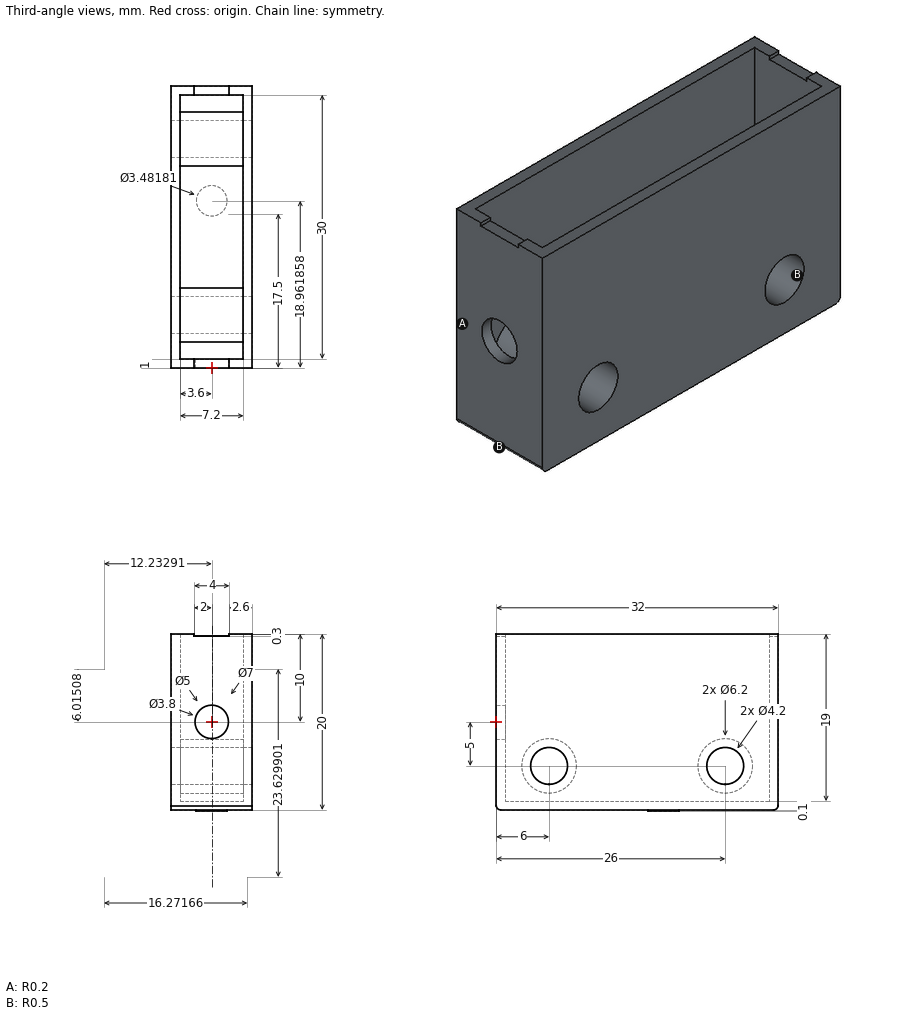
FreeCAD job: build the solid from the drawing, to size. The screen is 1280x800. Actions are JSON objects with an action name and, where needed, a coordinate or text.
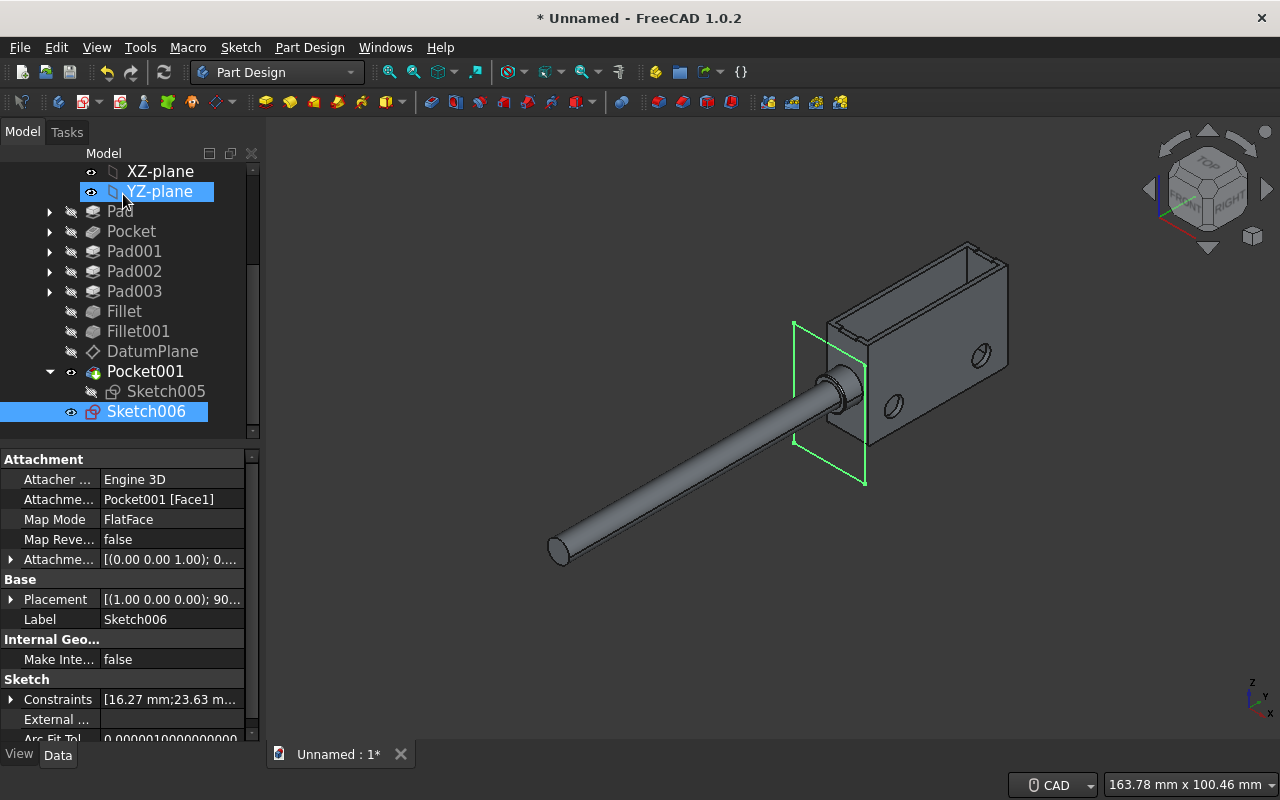
{"action": "left_click", "coordinate": [432, 102]}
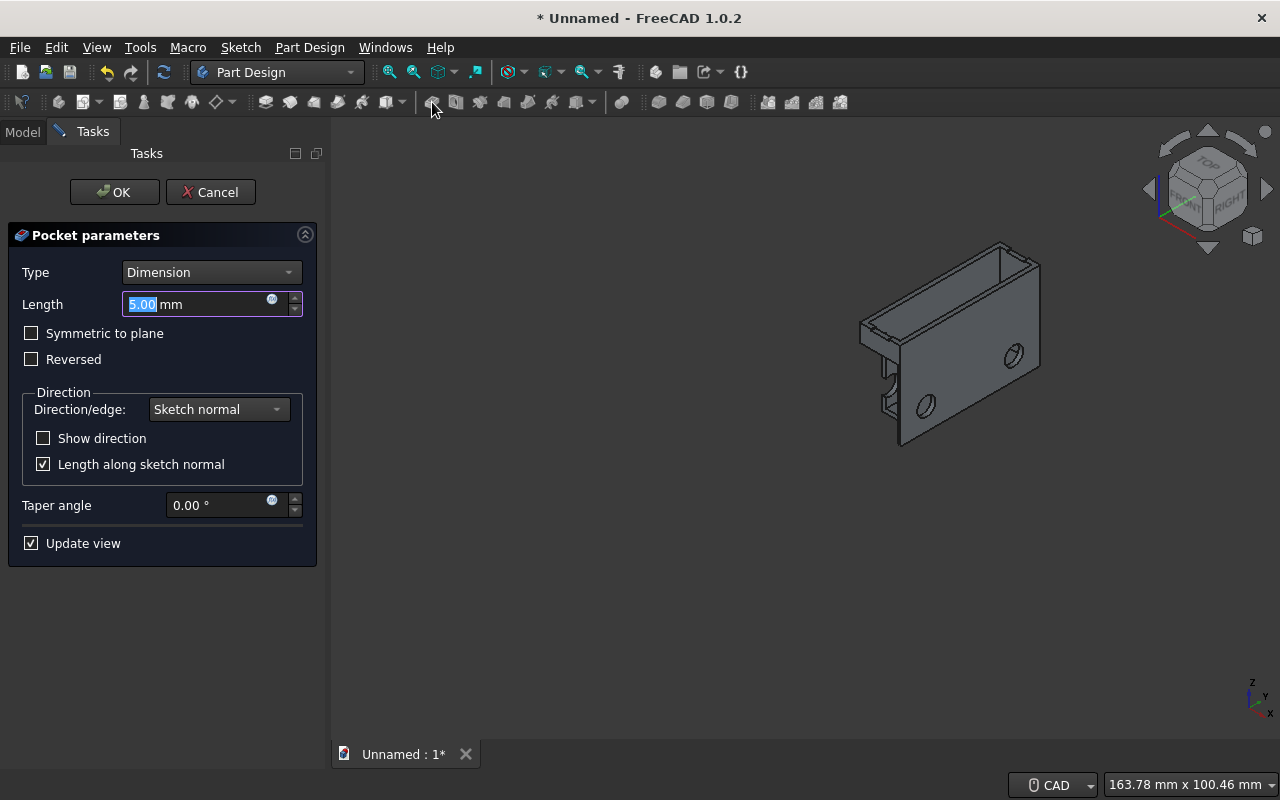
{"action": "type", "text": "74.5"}
{"action": "key", "text": "Tab"}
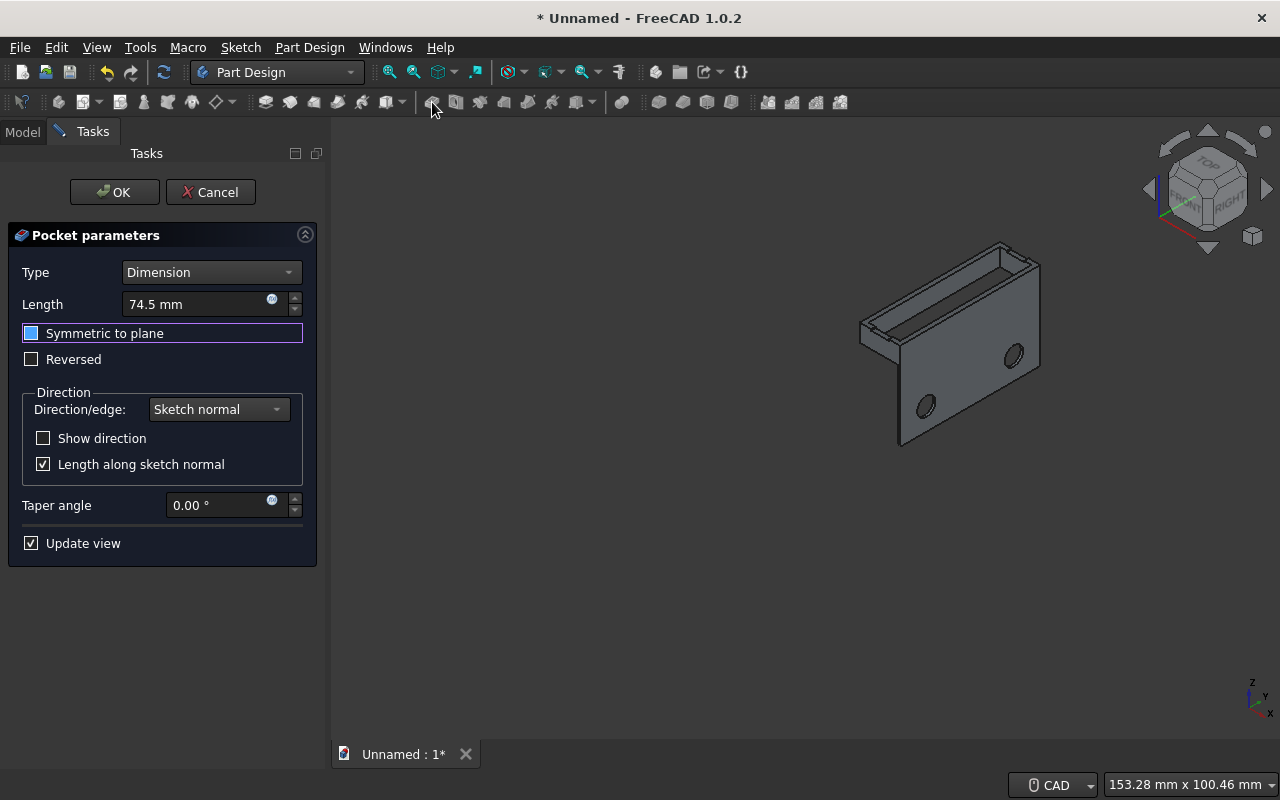
{"action": "left_click", "coordinate": [30, 359]}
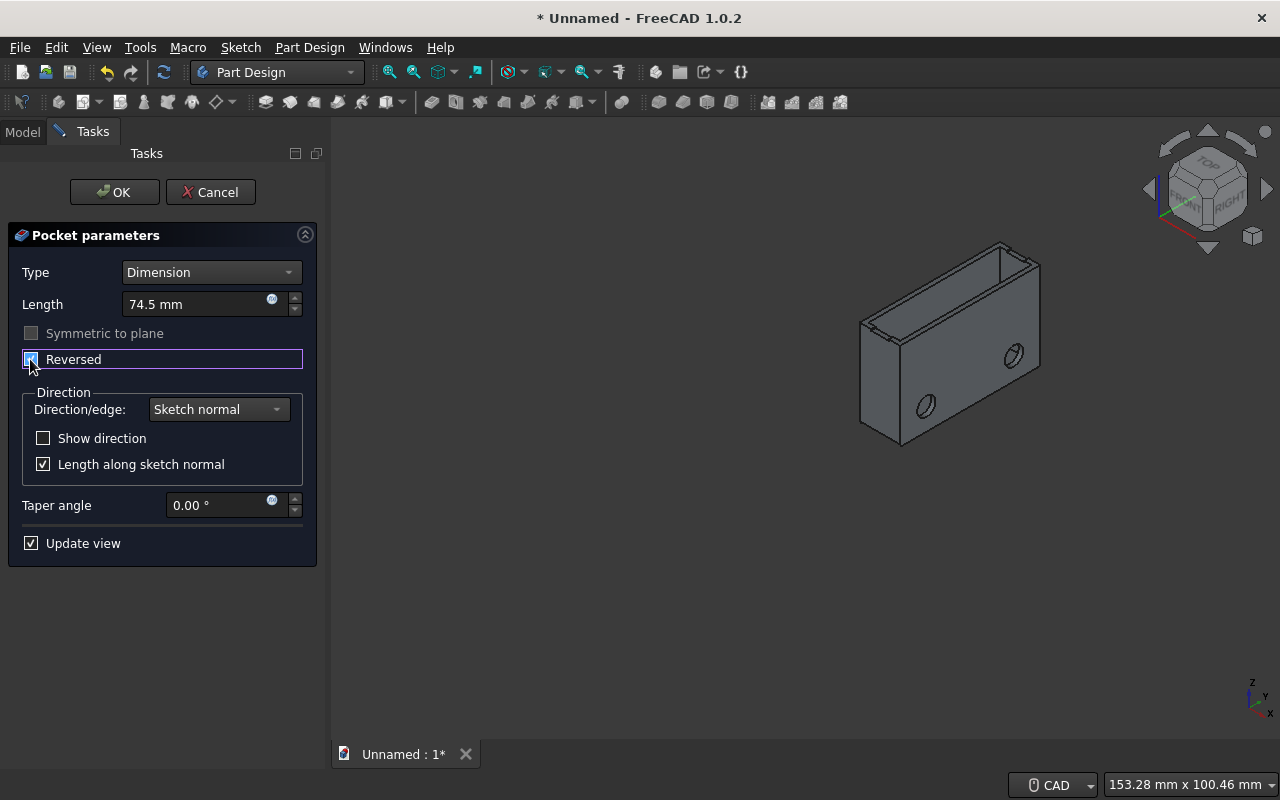
{"action": "left_click", "coordinate": [115, 192]}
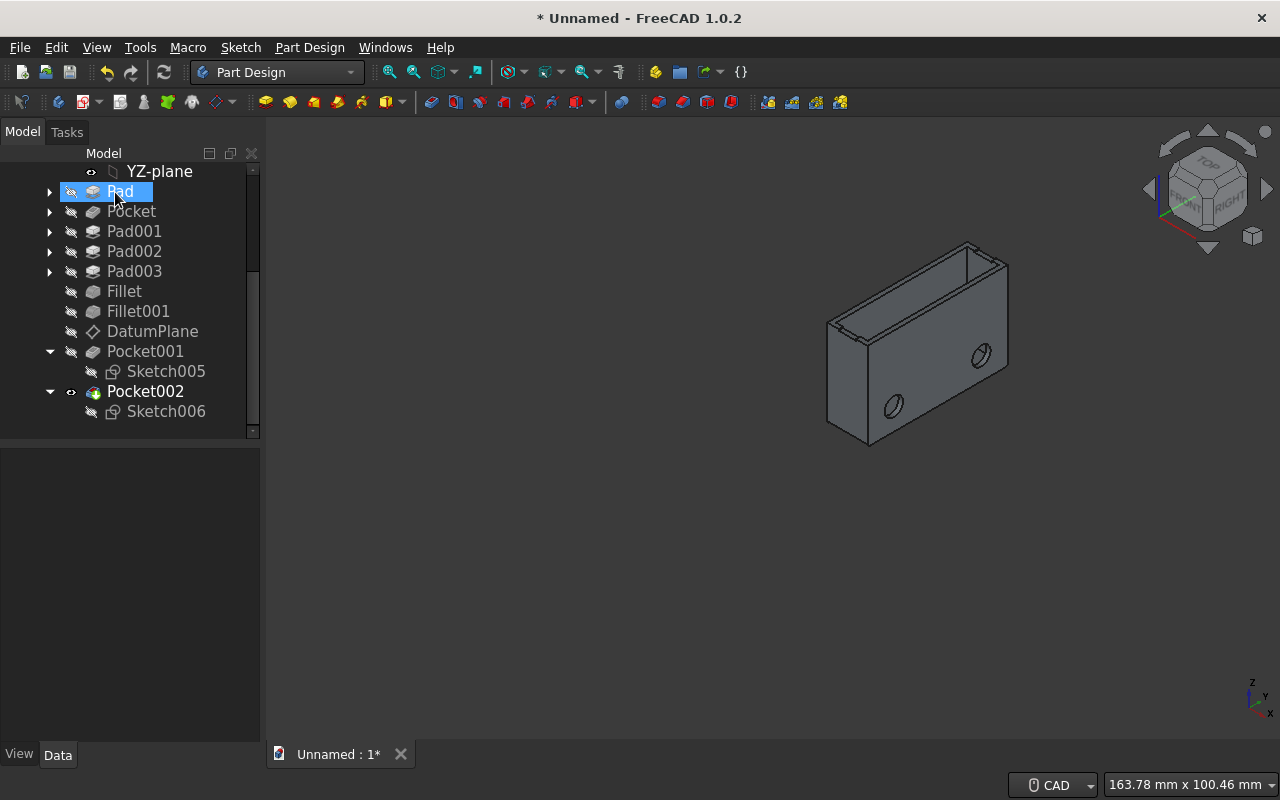
{"action": "left_click", "coordinate": [390, 72]}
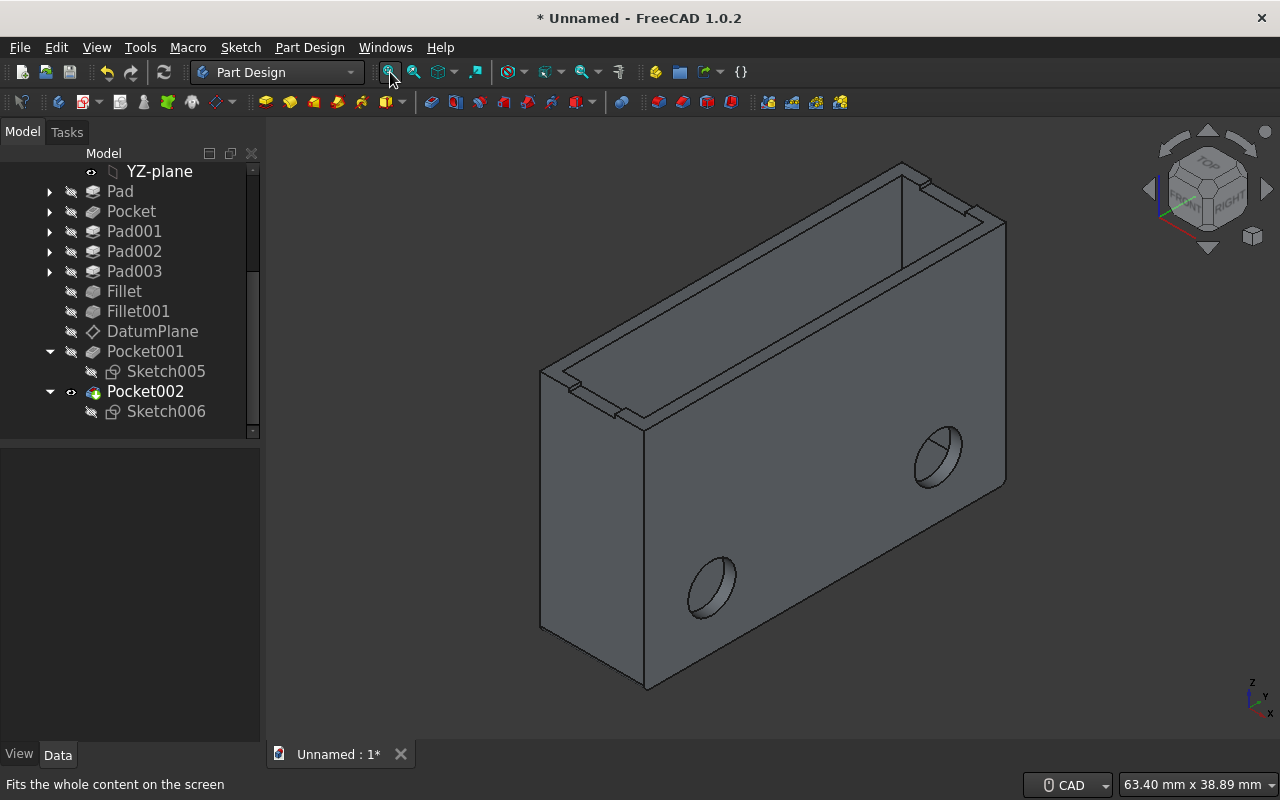
{"action": "left_click", "coordinate": [592, 491]}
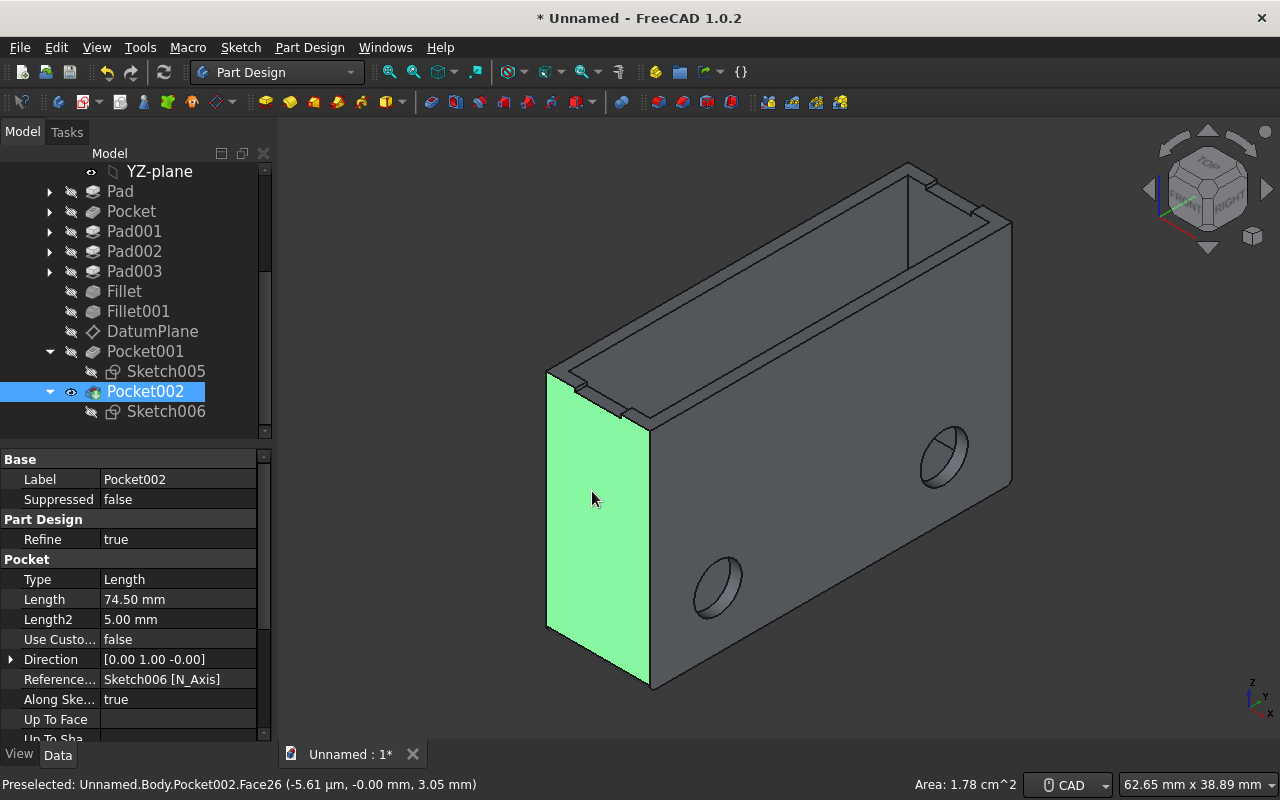
{"action": "left_click", "coordinate": [84, 102]}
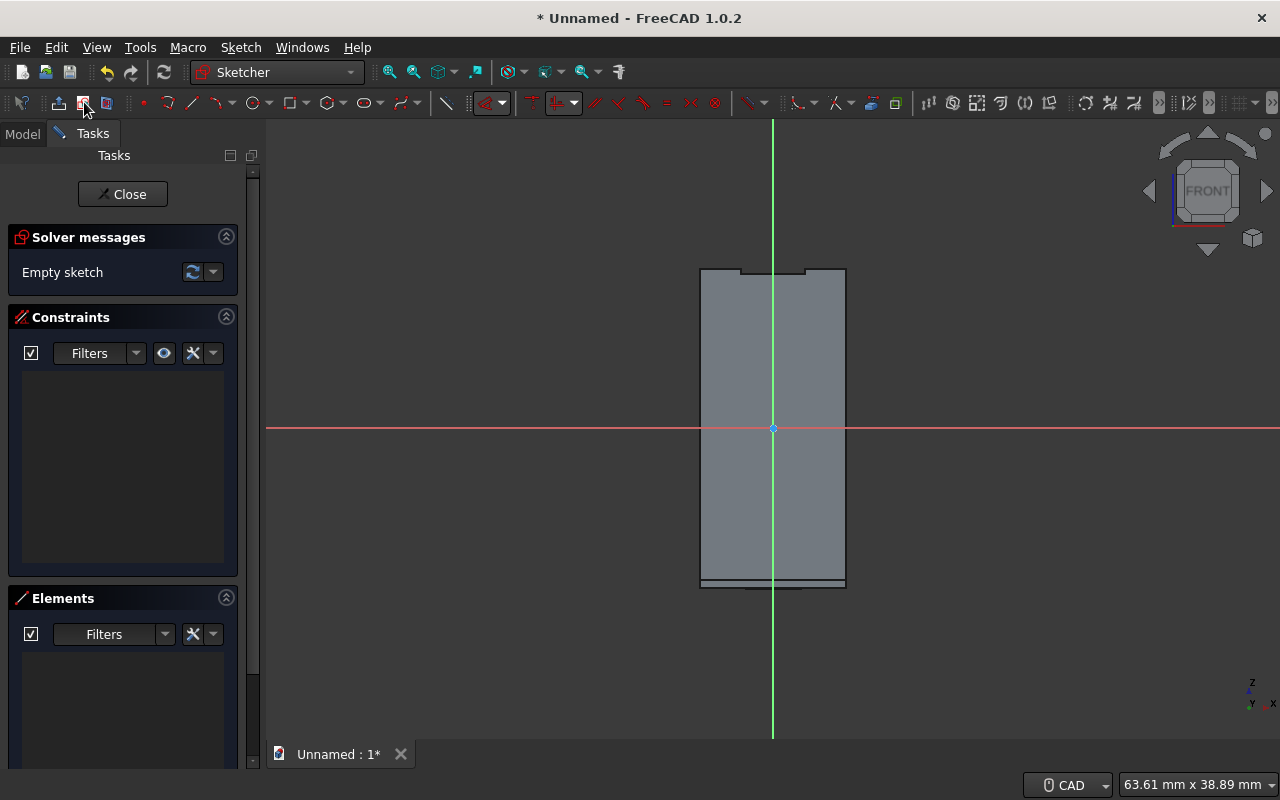
{"action": "scroll", "coordinate": [787, 428], "scroll_direction": "up", "scroll_amount": 9}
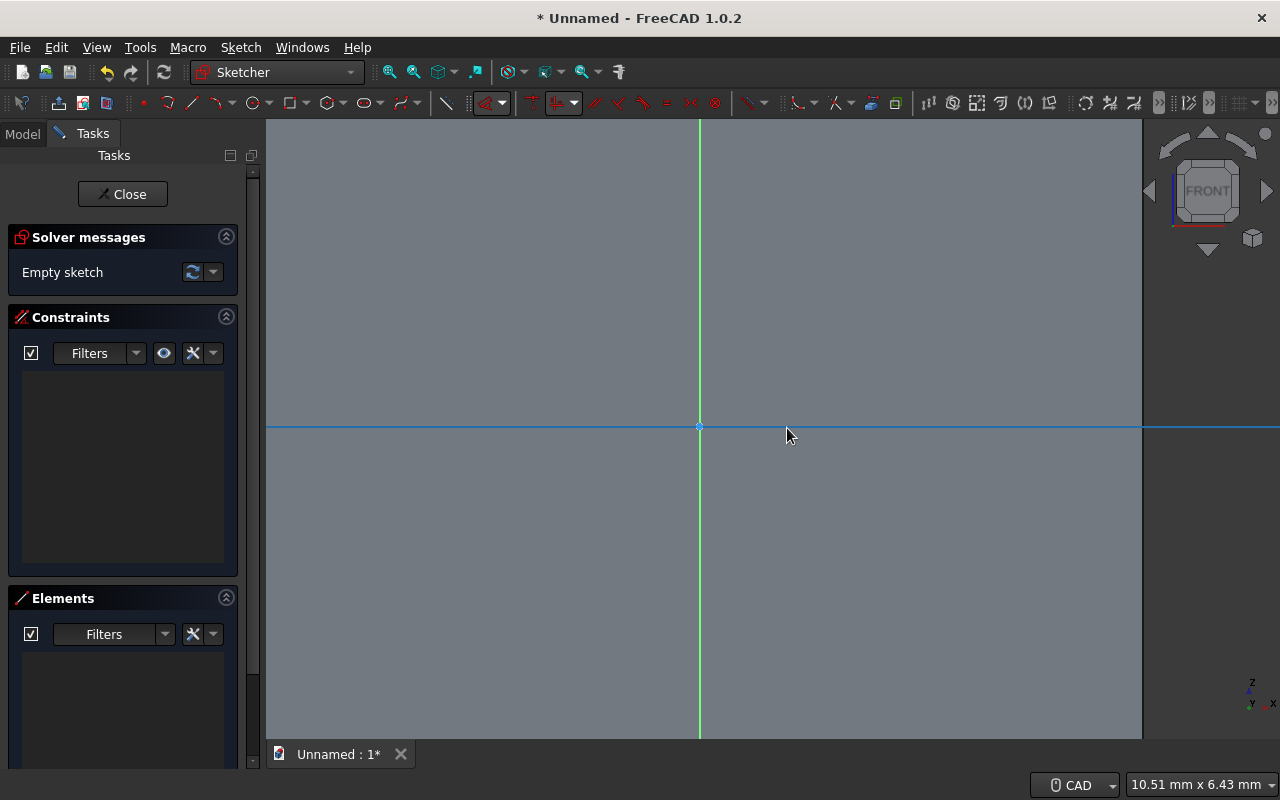
{"action": "left_click", "coordinate": [254, 104]}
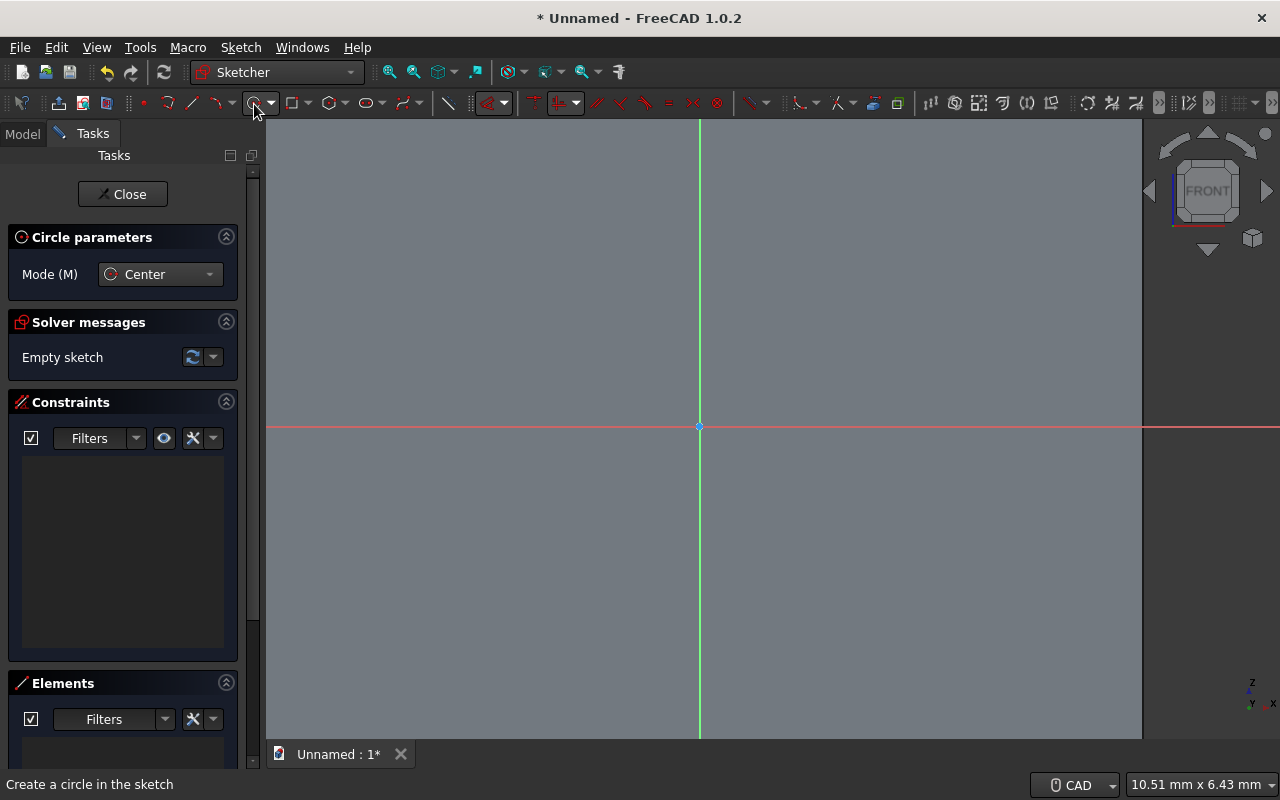
{"action": "left_click", "coordinate": [700, 427]}
{"action": "mouse_move", "coordinate": [829, 297]}